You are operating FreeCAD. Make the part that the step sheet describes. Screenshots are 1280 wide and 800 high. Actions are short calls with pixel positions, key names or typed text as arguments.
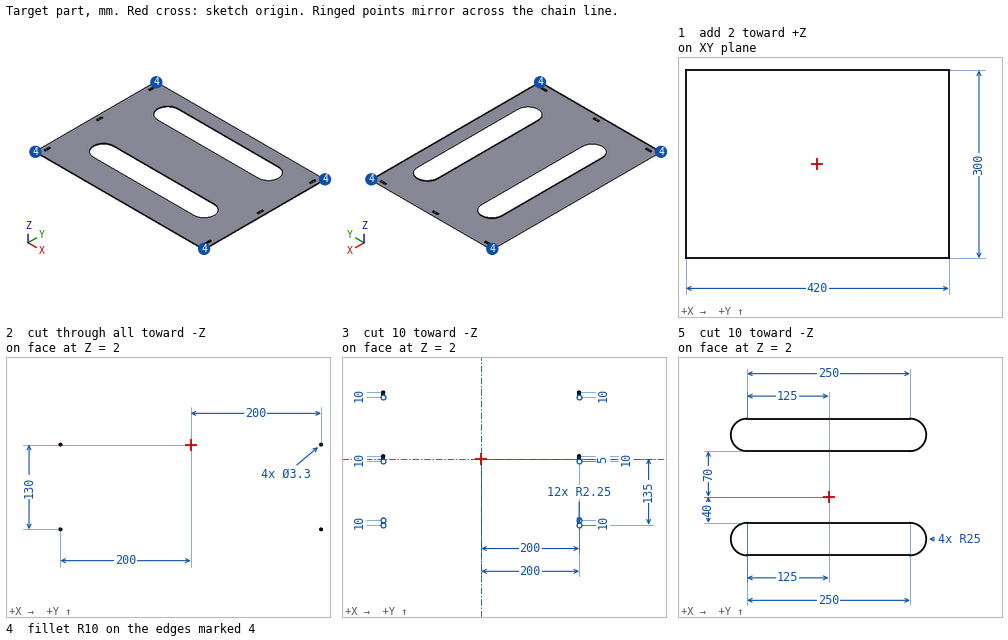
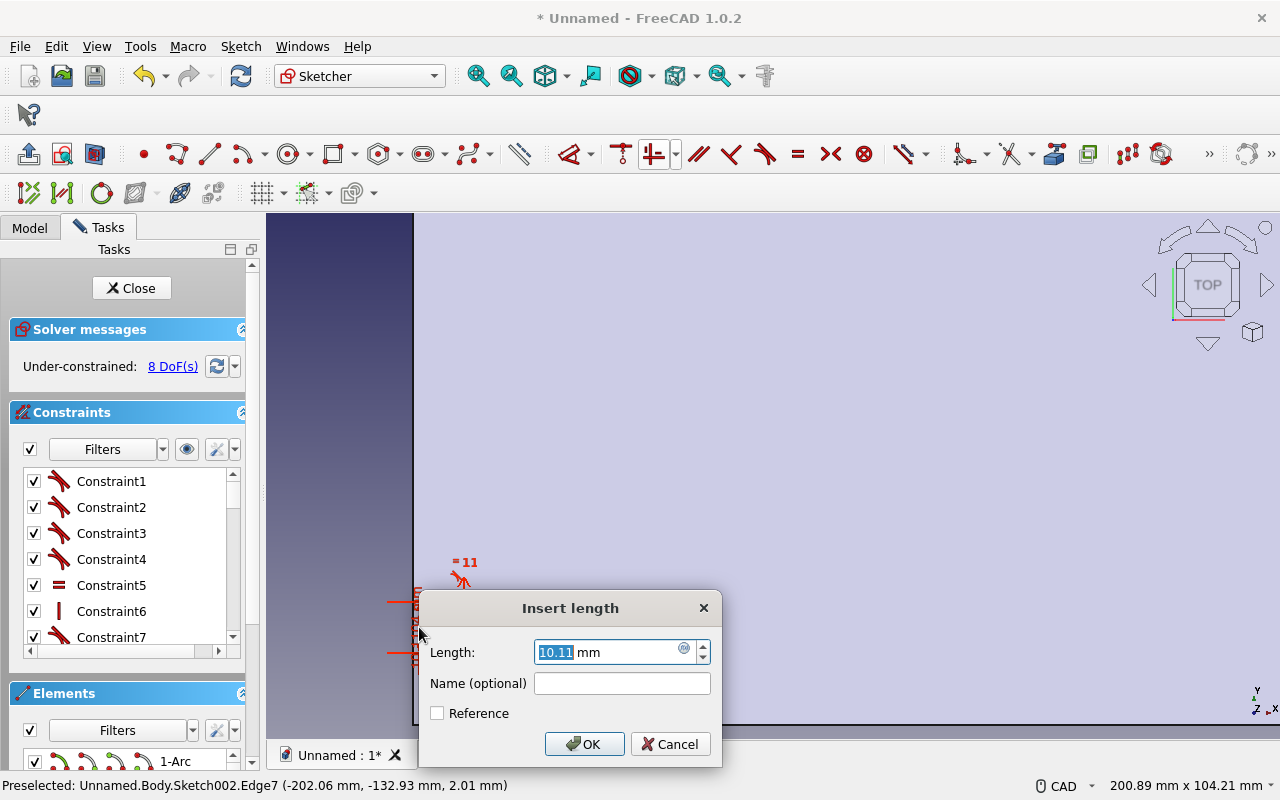
text(10)
key(Return)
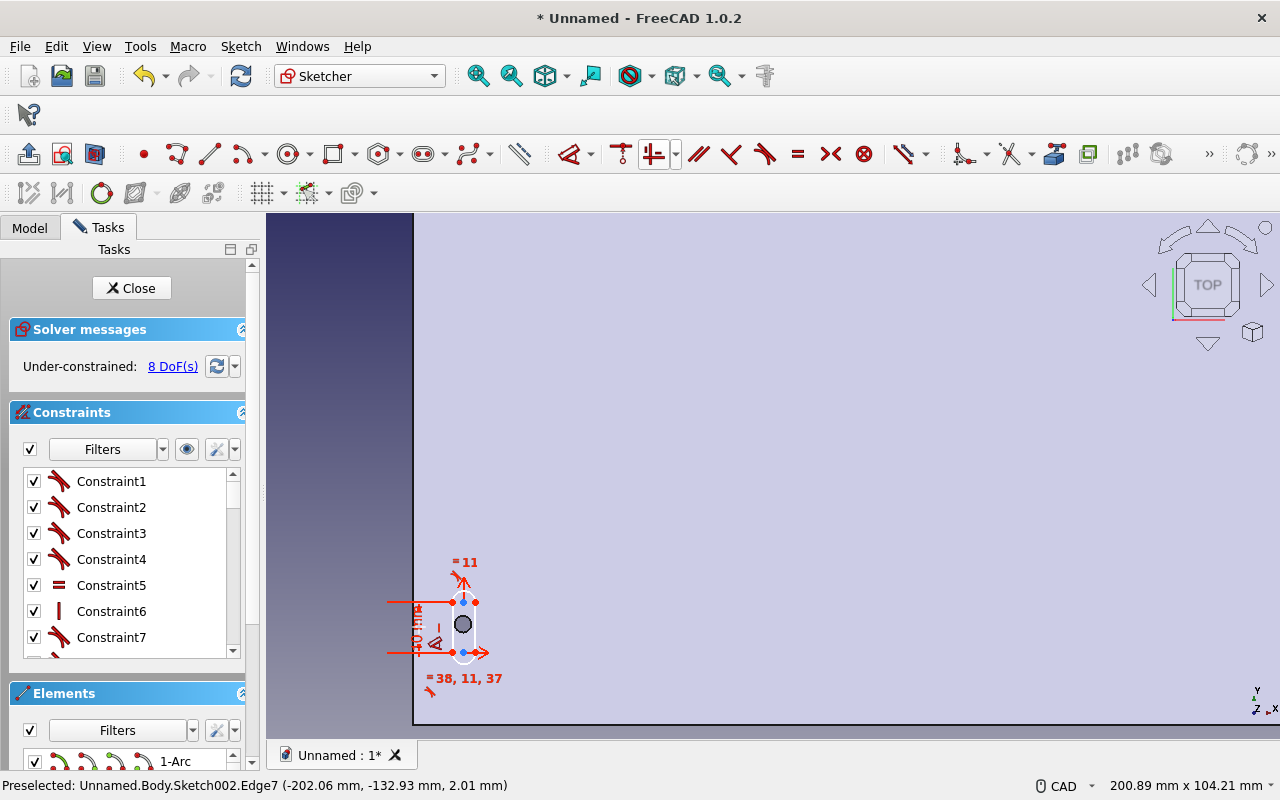
scroll(453, 642, down, 7)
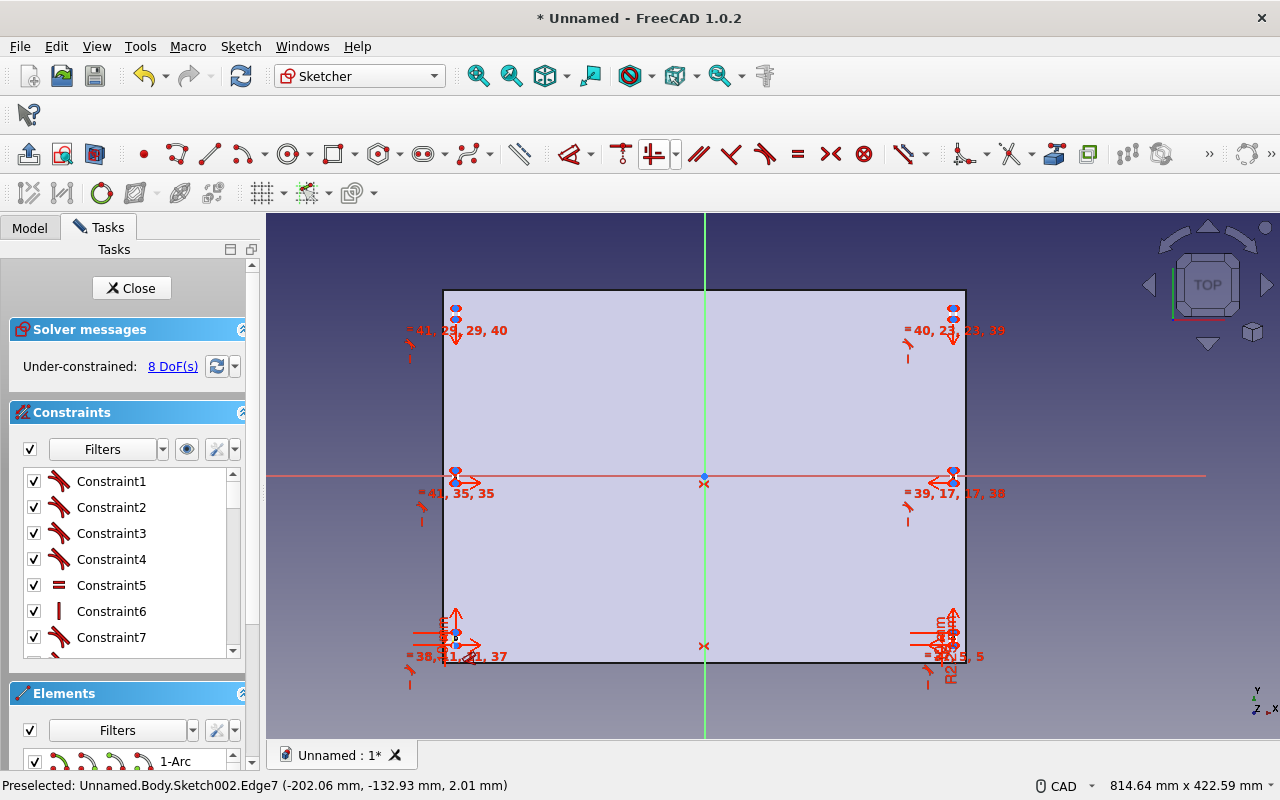
scroll(951, 479, up, 8)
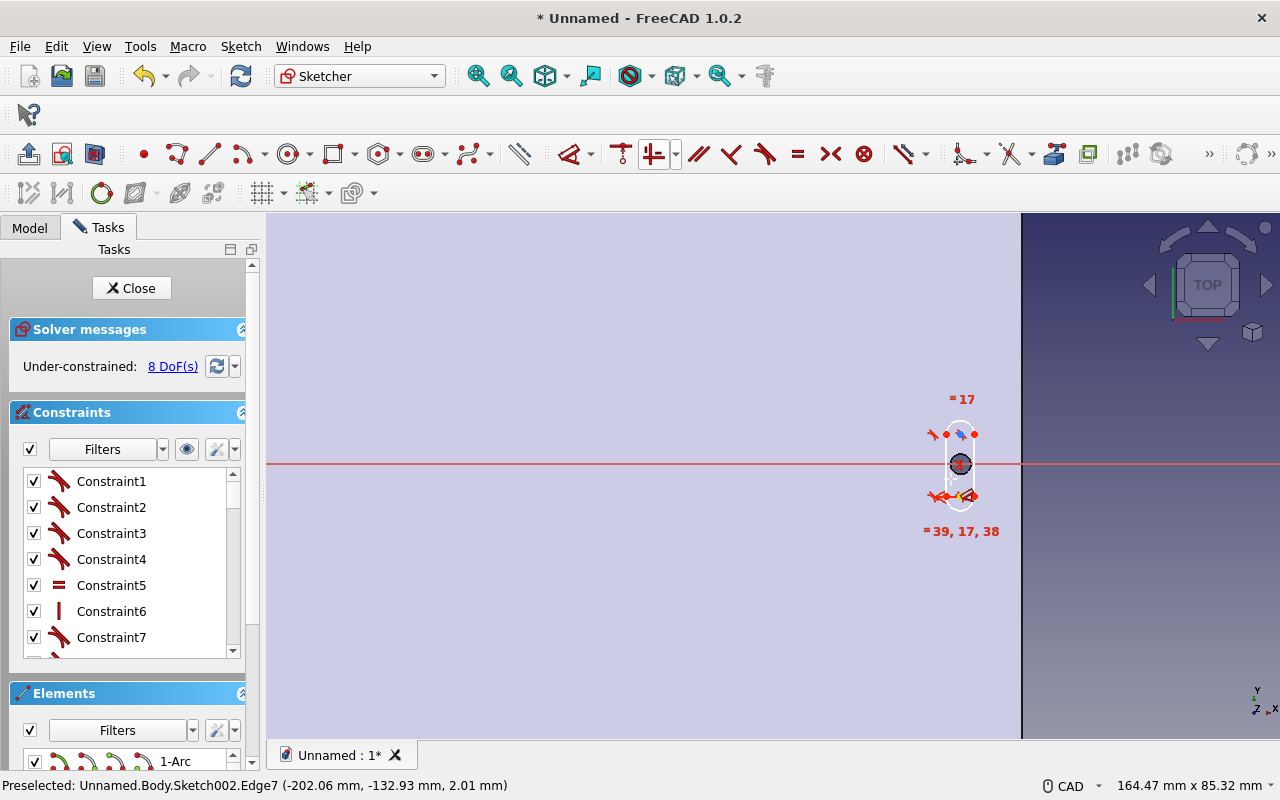
click(946, 478)
click(912, 480)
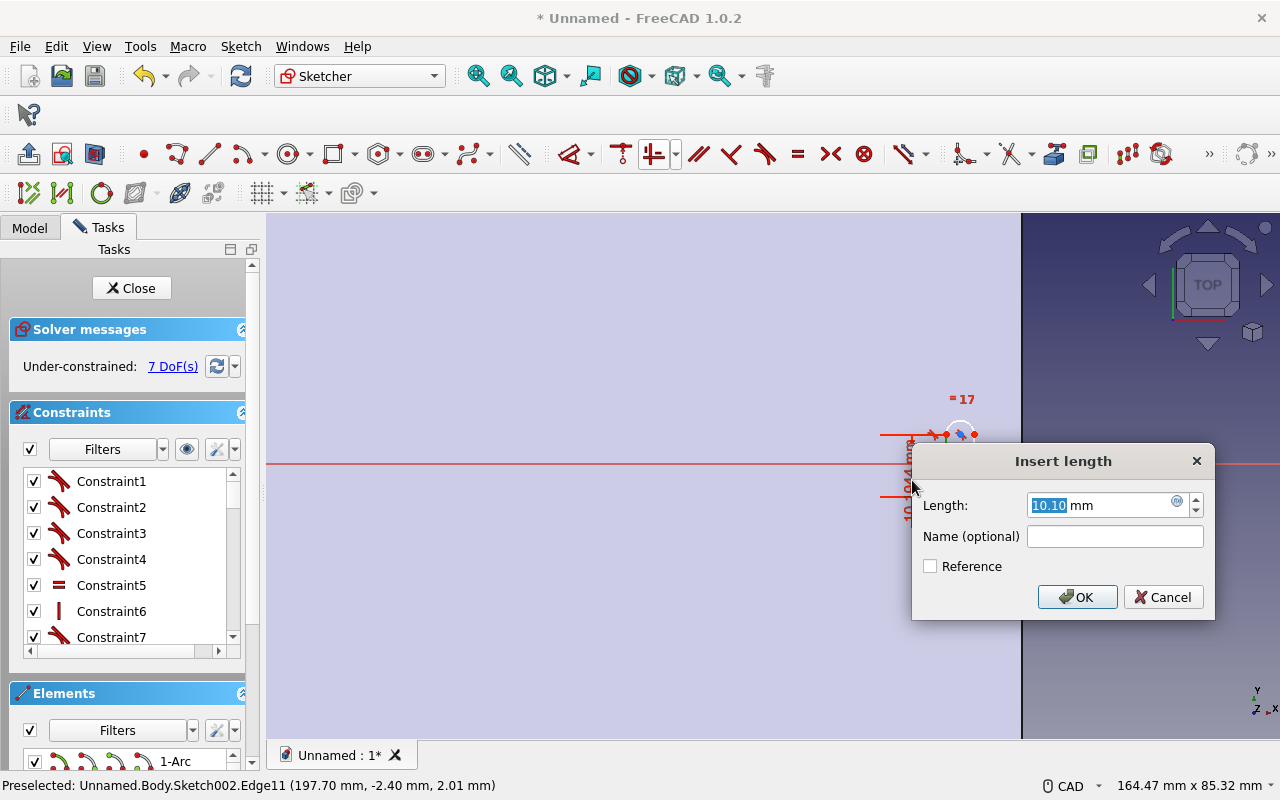
text(10)
key(Return)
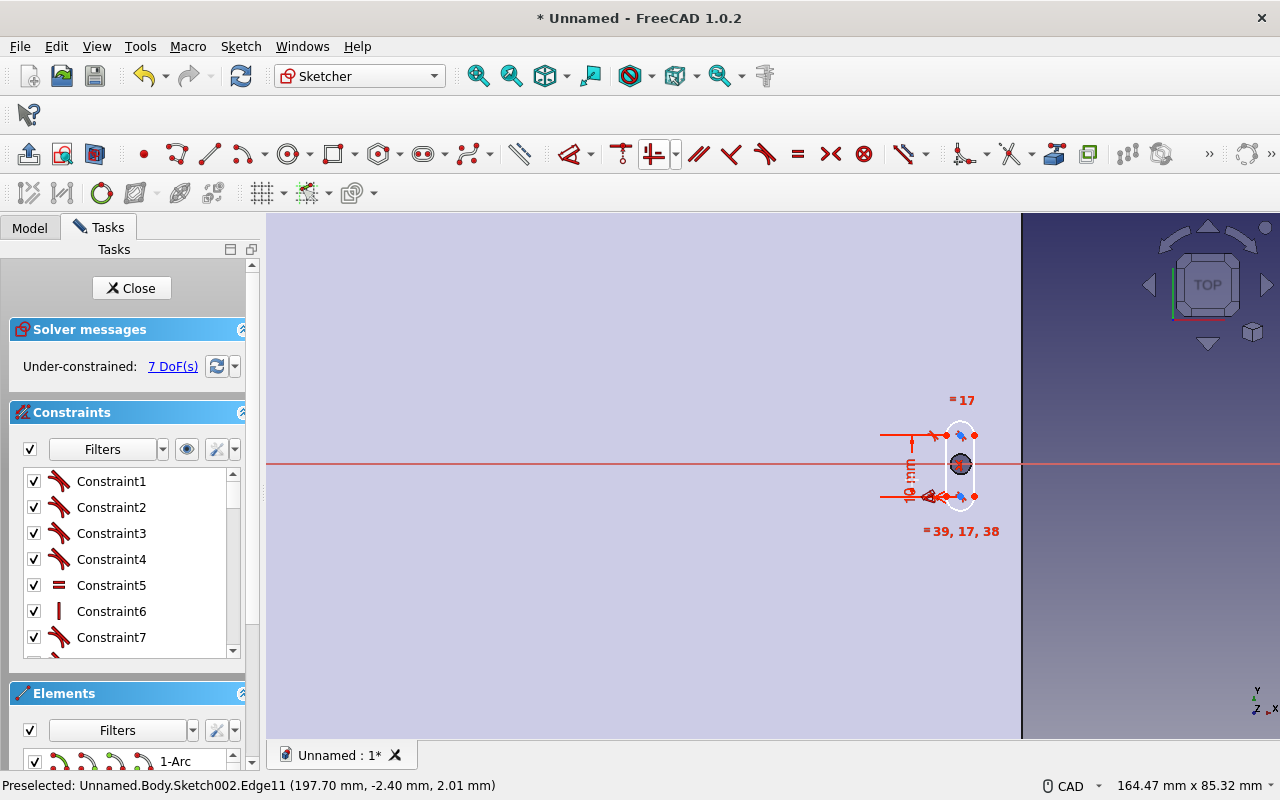
scroll(952, 479, down, 8)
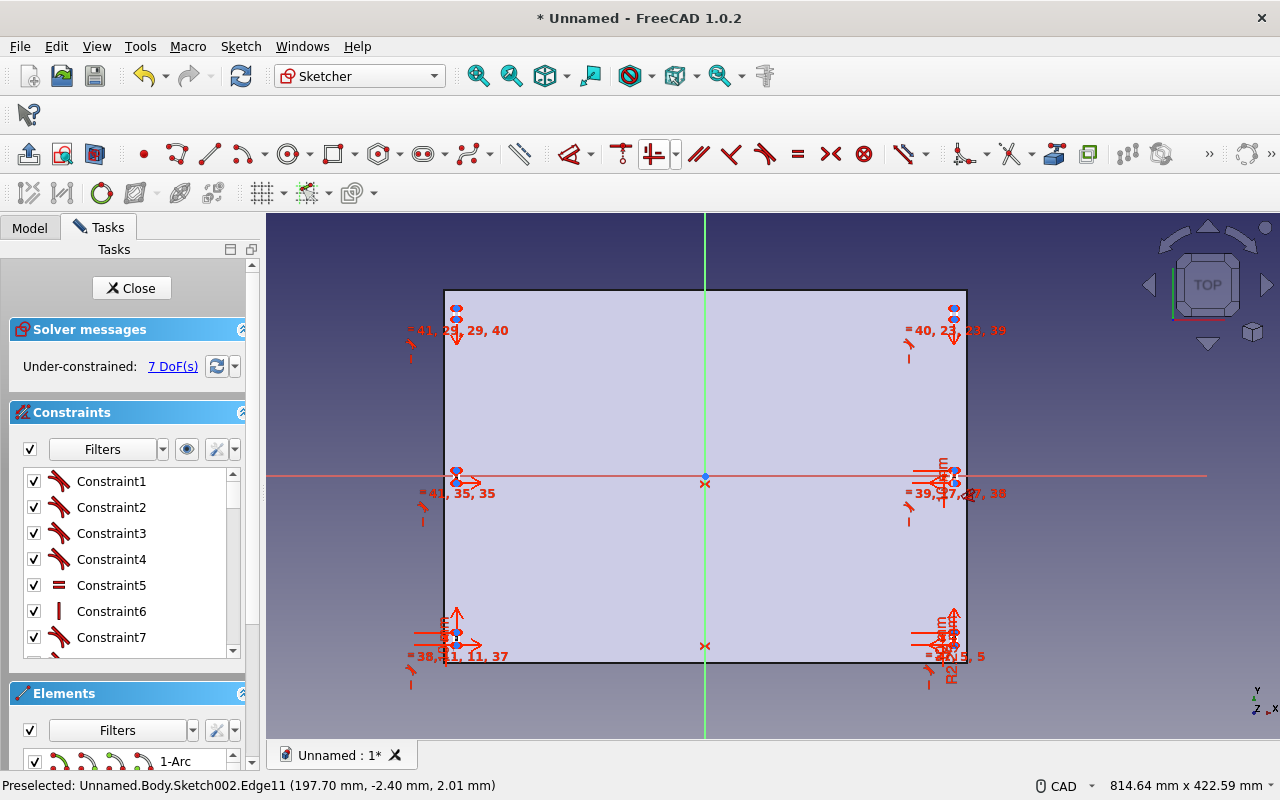
scroll(951, 317, up, 8)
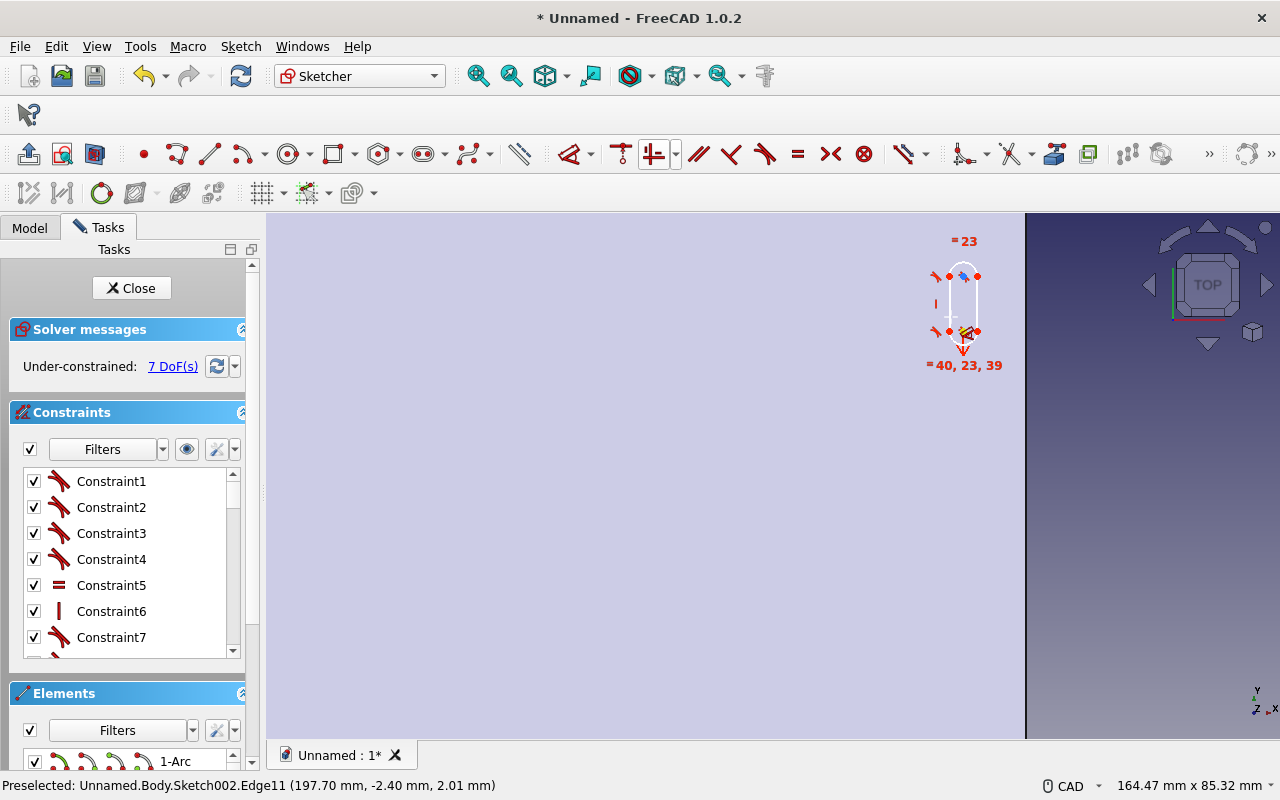
click(950, 315)
click(916, 304)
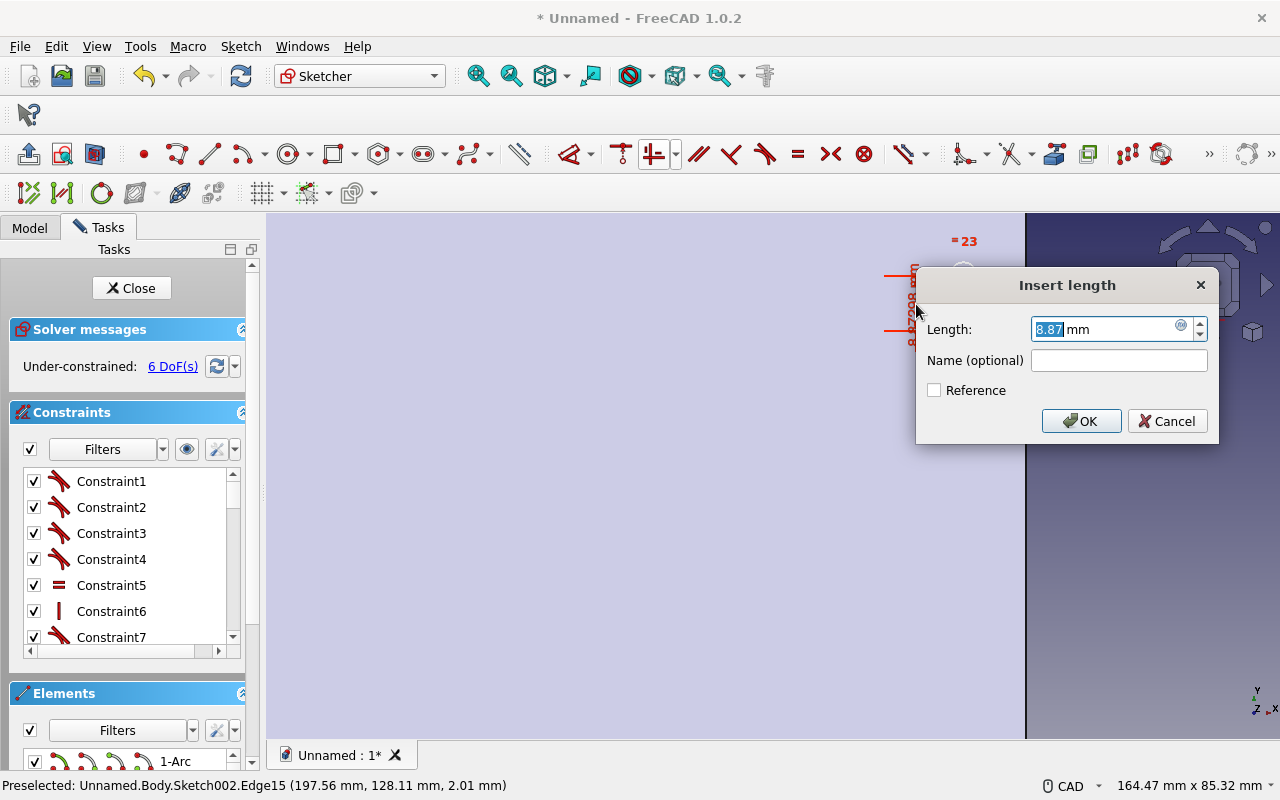
text(10)
key(Return)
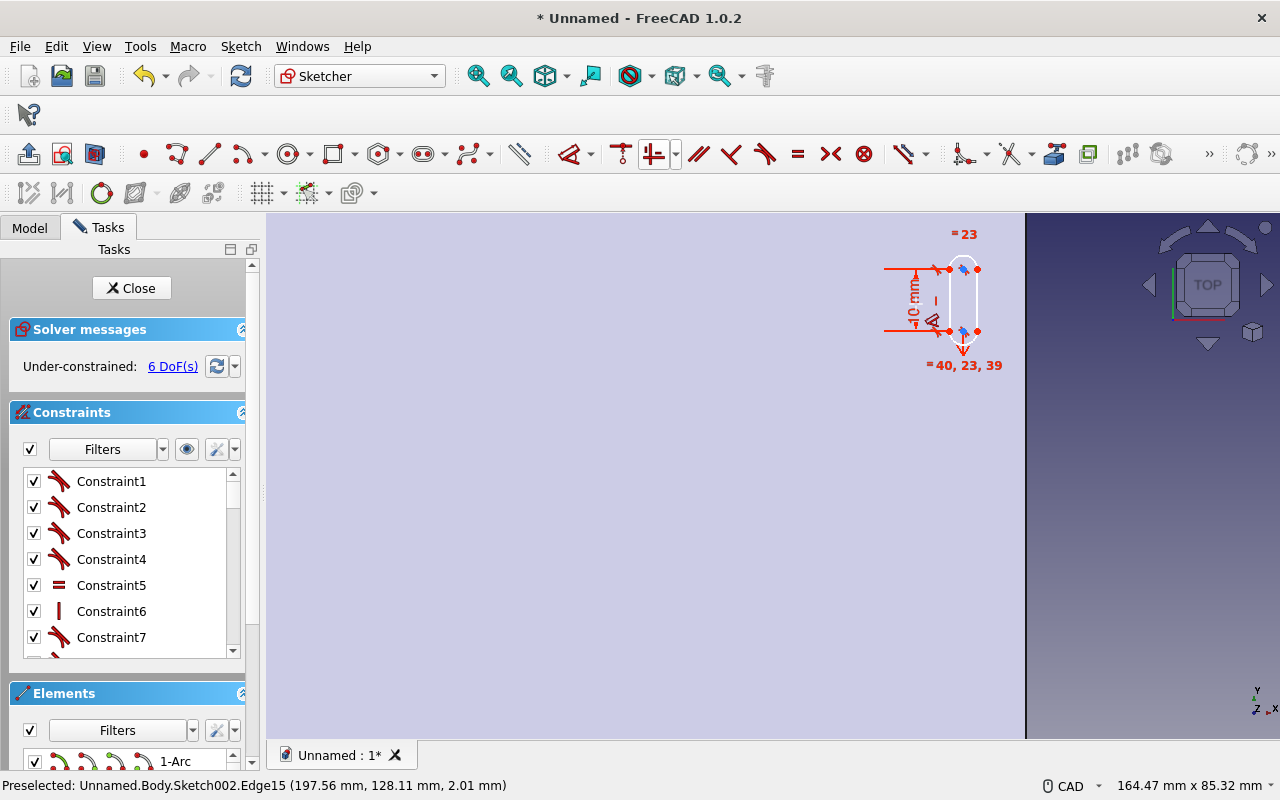
scroll(951, 317, down, 8)